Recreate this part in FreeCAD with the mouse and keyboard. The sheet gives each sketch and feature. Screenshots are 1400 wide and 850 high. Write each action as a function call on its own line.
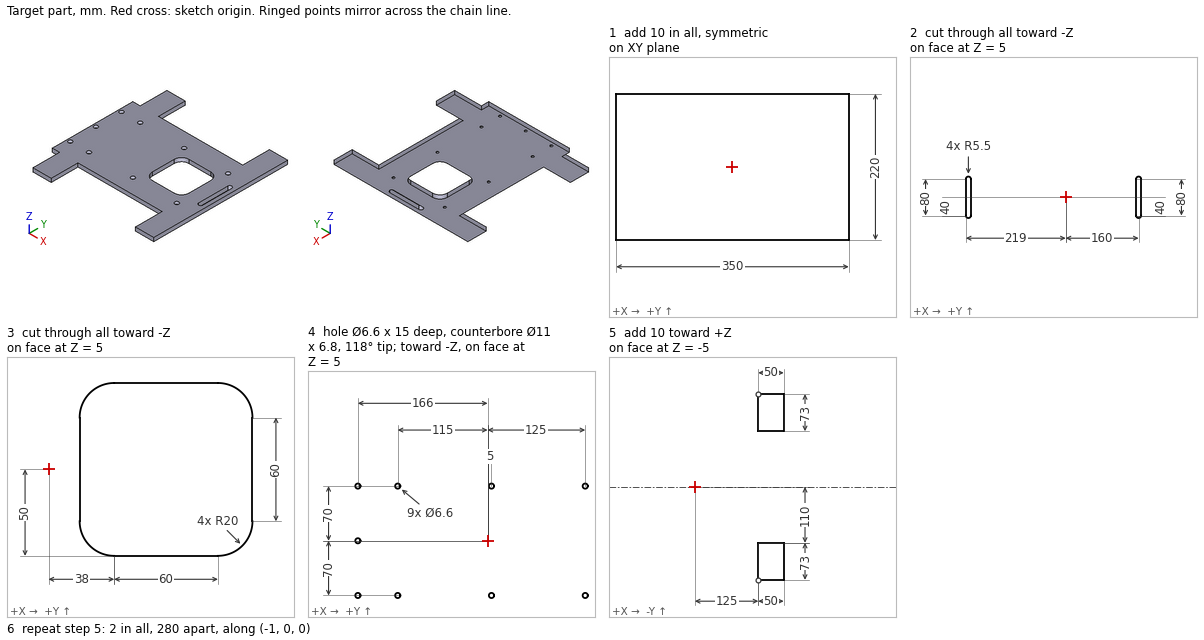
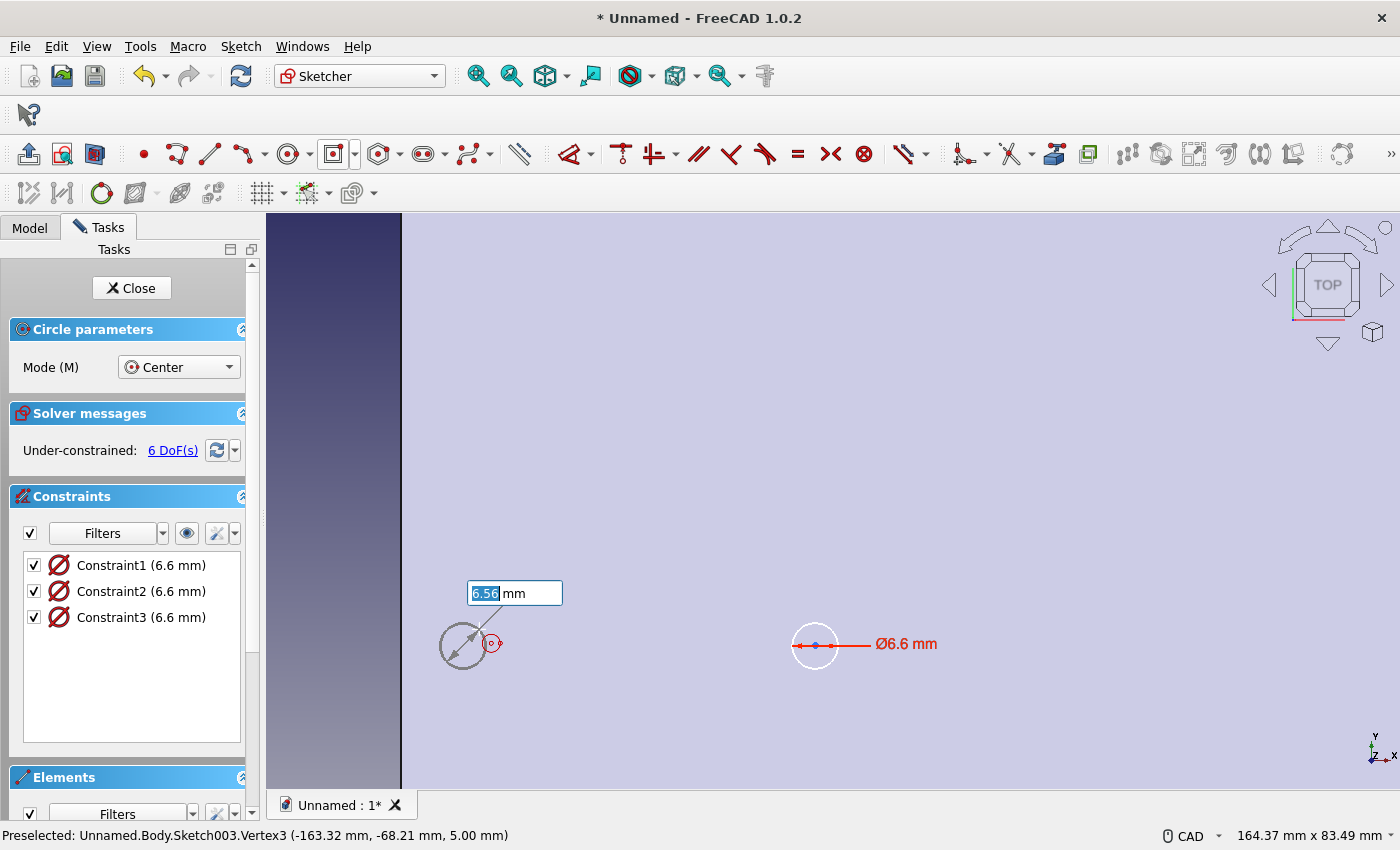
text(6.6)
key(Return)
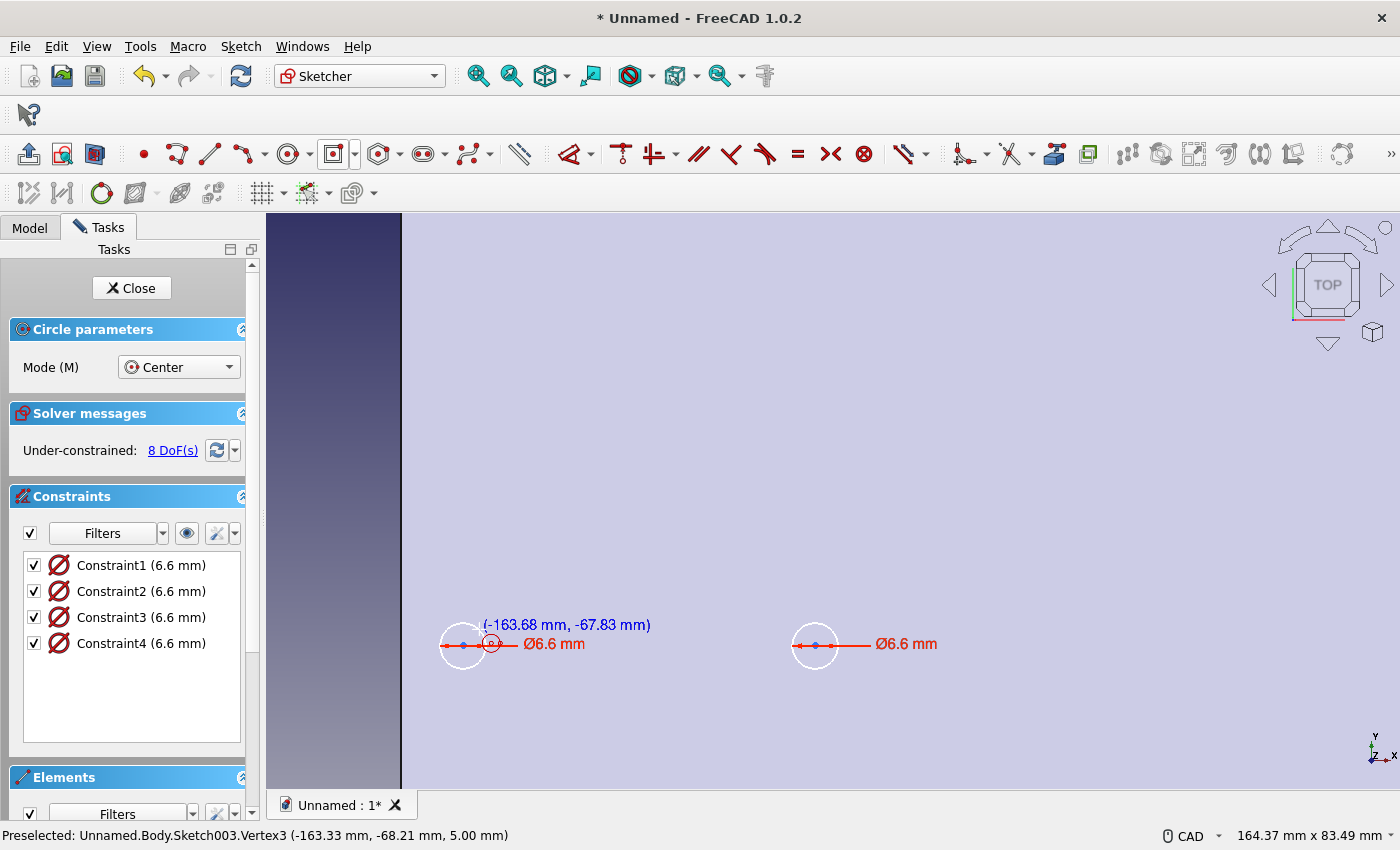
scroll(462, 647, down, 6)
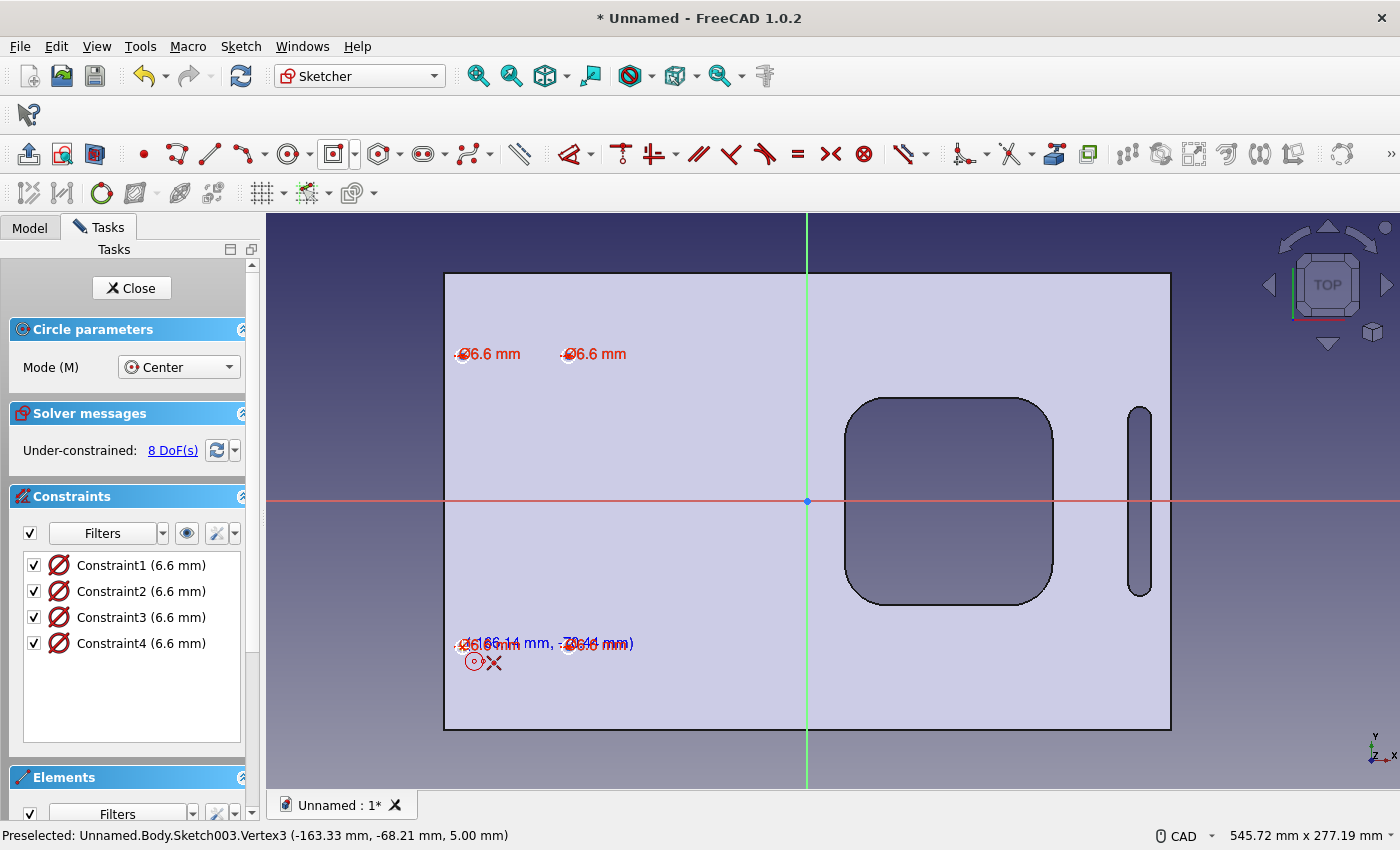
scroll(462, 501, up, 6)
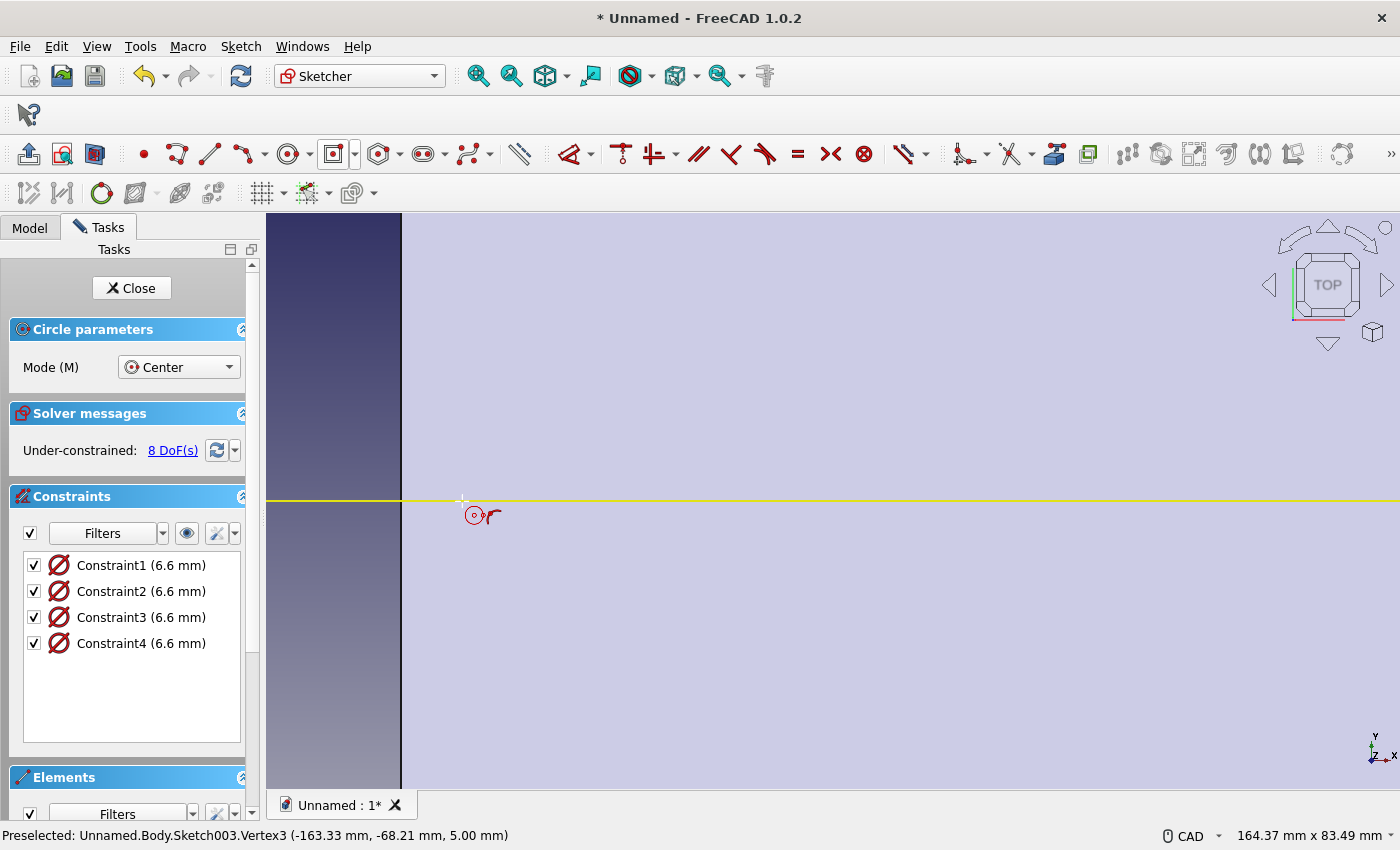
click(463, 501)
move(479, 485)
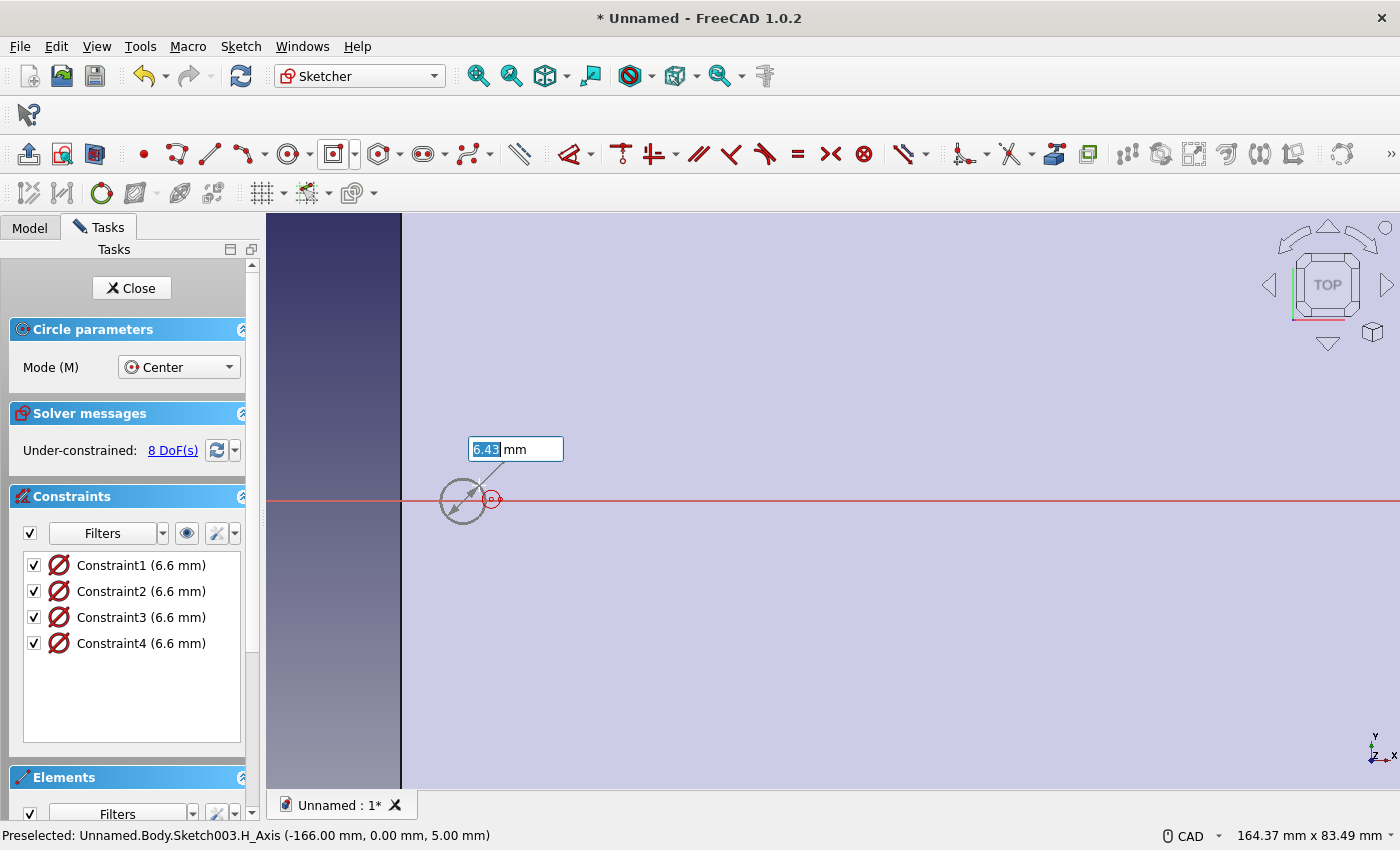
text(6.6)
key(Return)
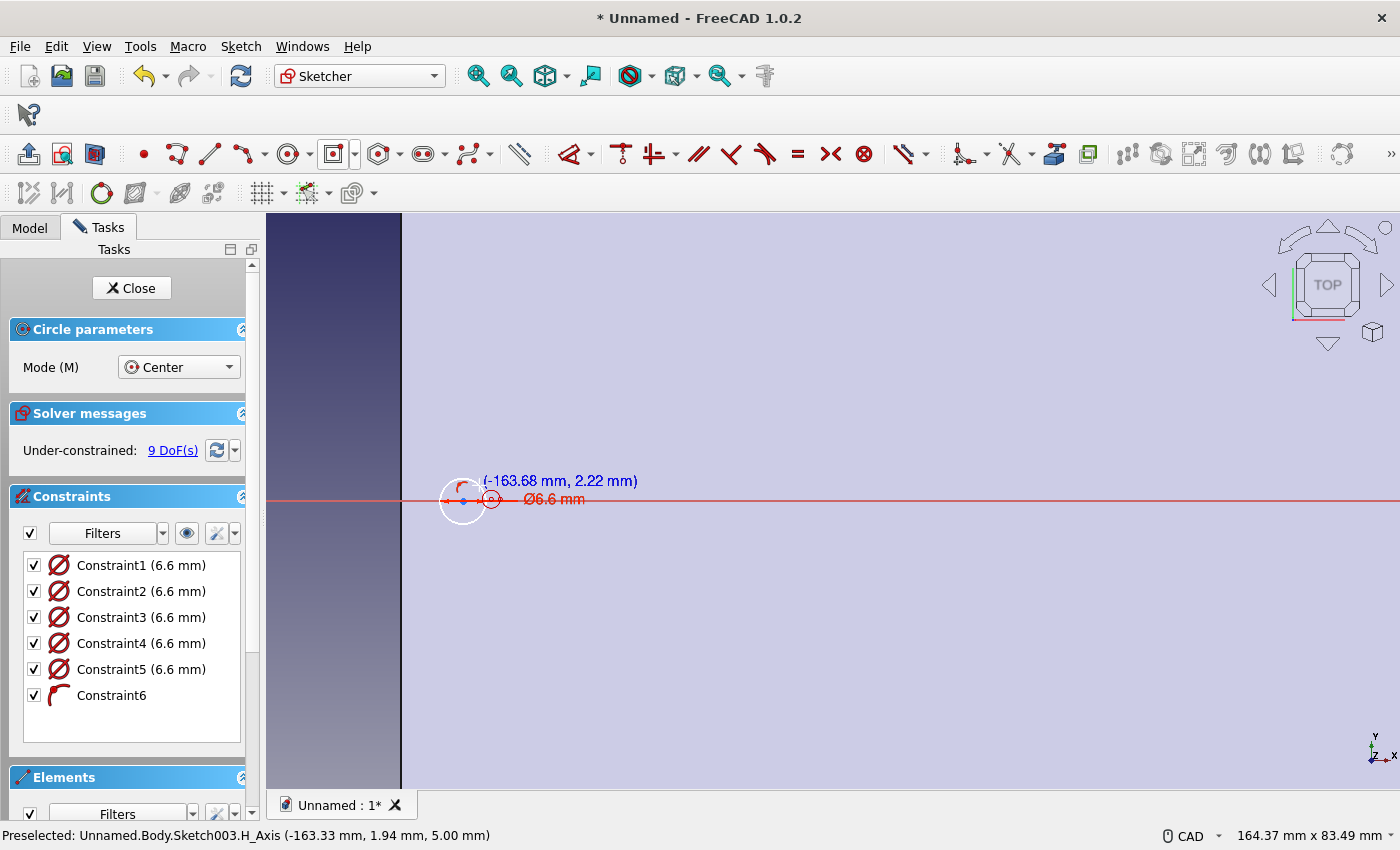
scroll(462, 501, down, 6)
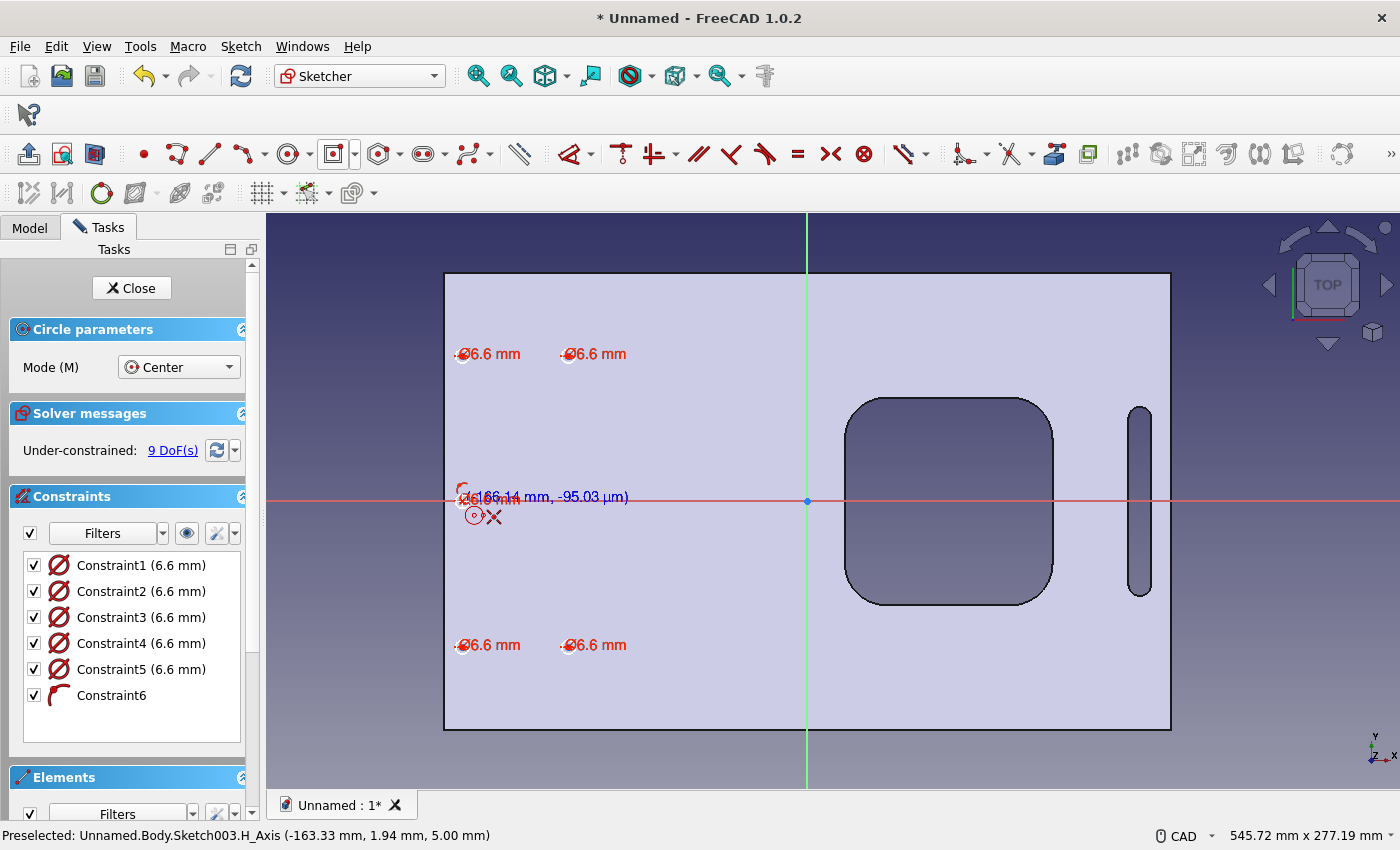
scroll(818, 356, up, 6)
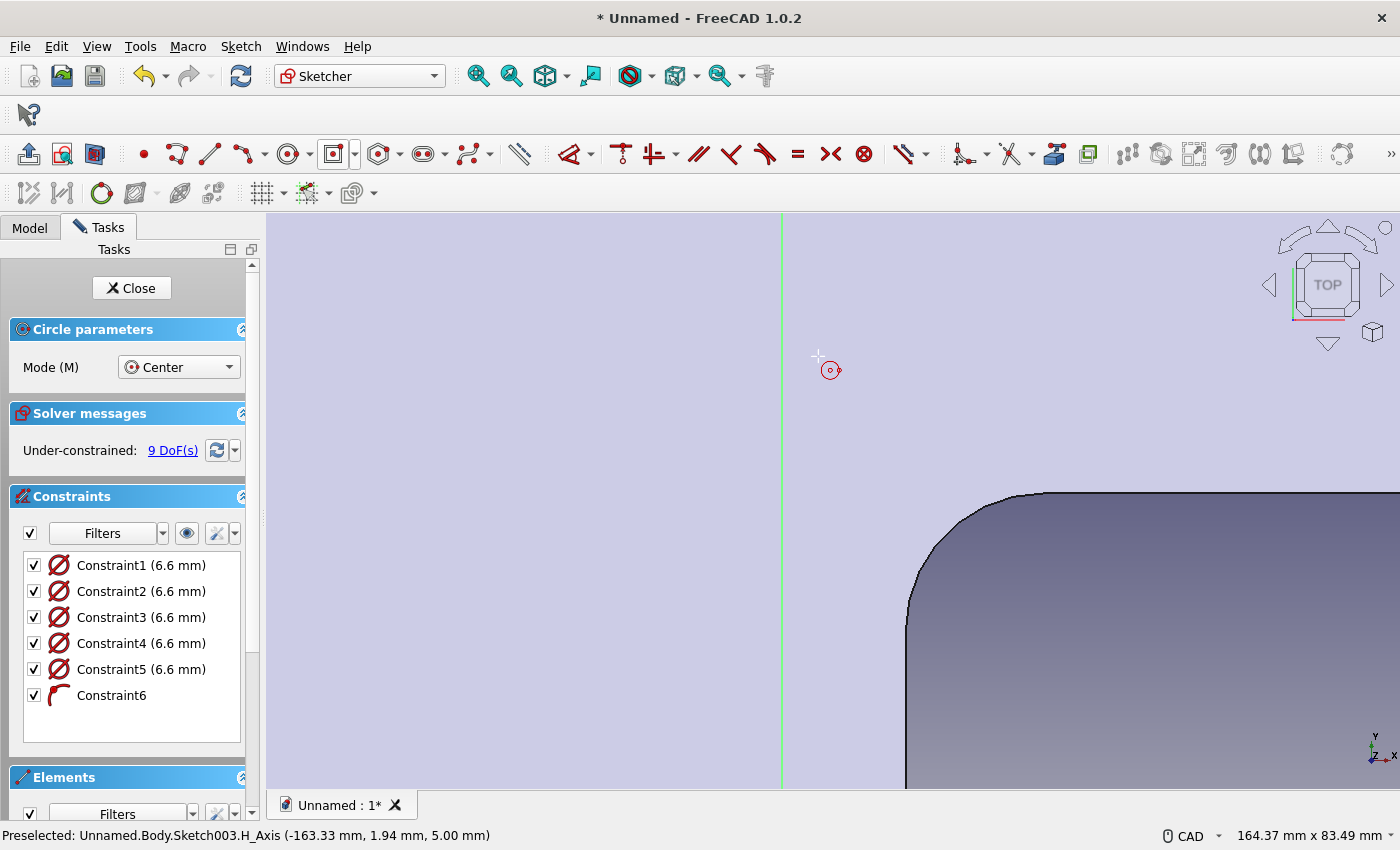
click(816, 355)
move(832, 339)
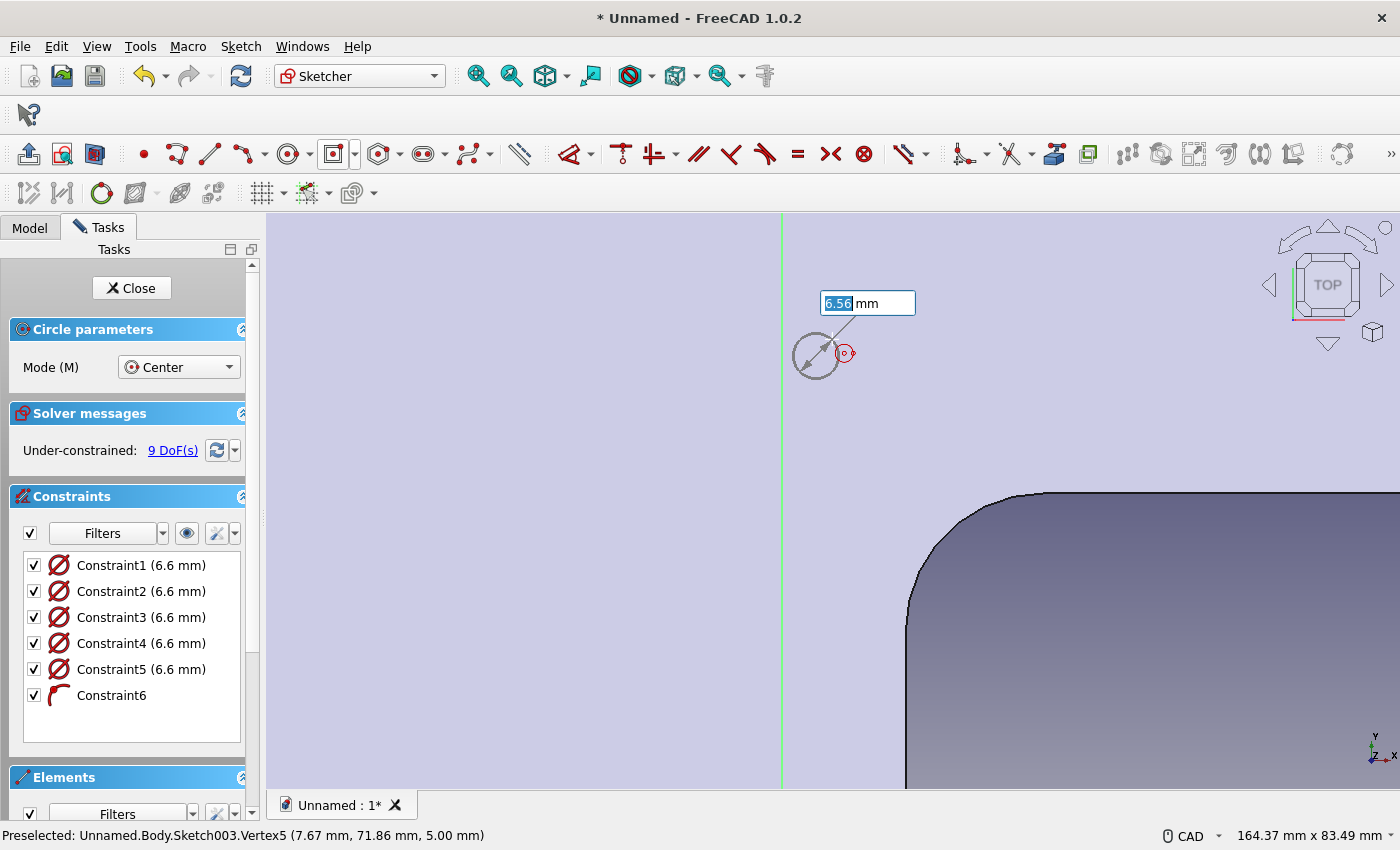
text(6.6)
key(Return)